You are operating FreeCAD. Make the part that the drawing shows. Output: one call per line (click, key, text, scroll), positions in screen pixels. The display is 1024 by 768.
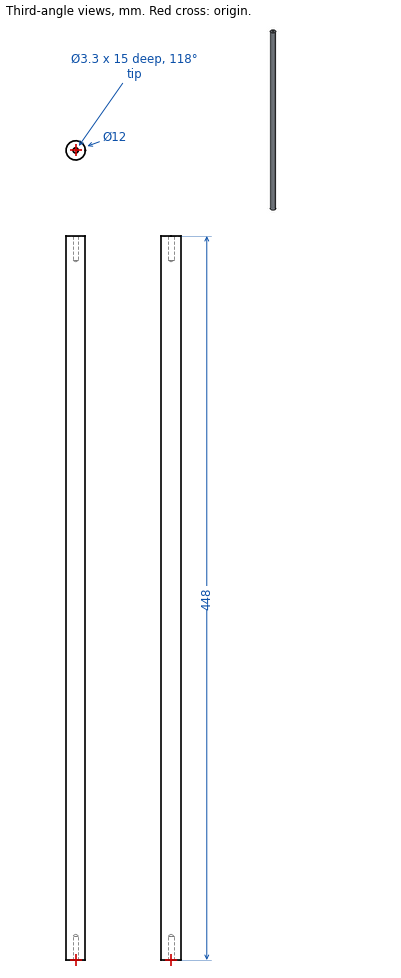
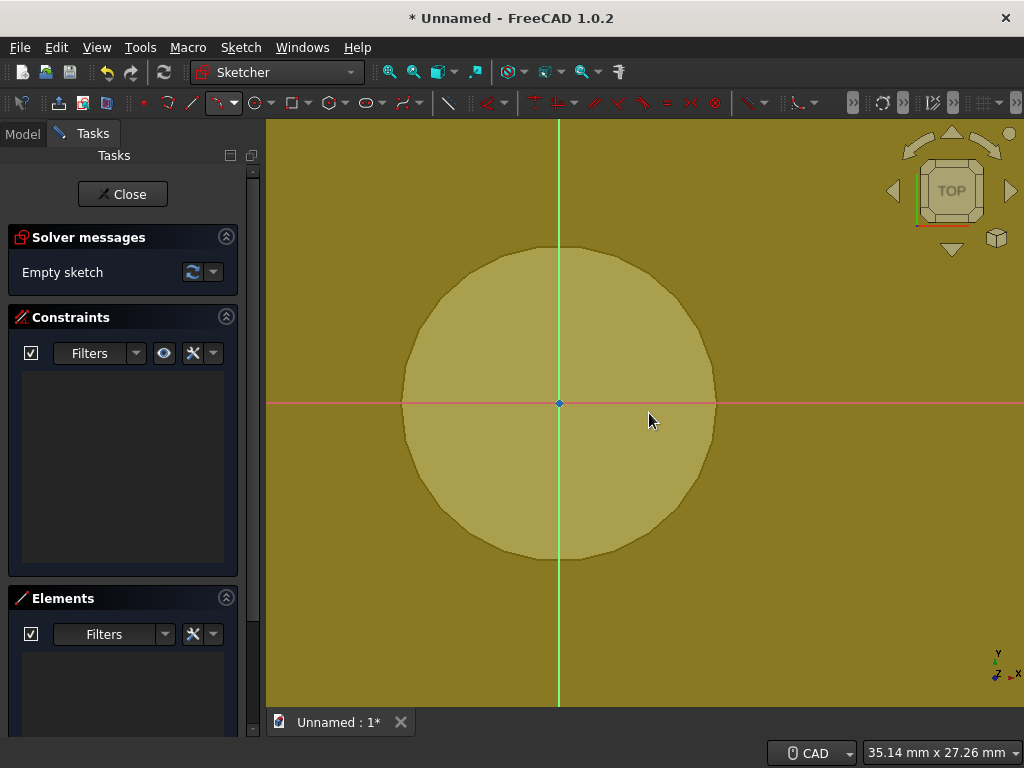
scroll(553, 400, up, 7)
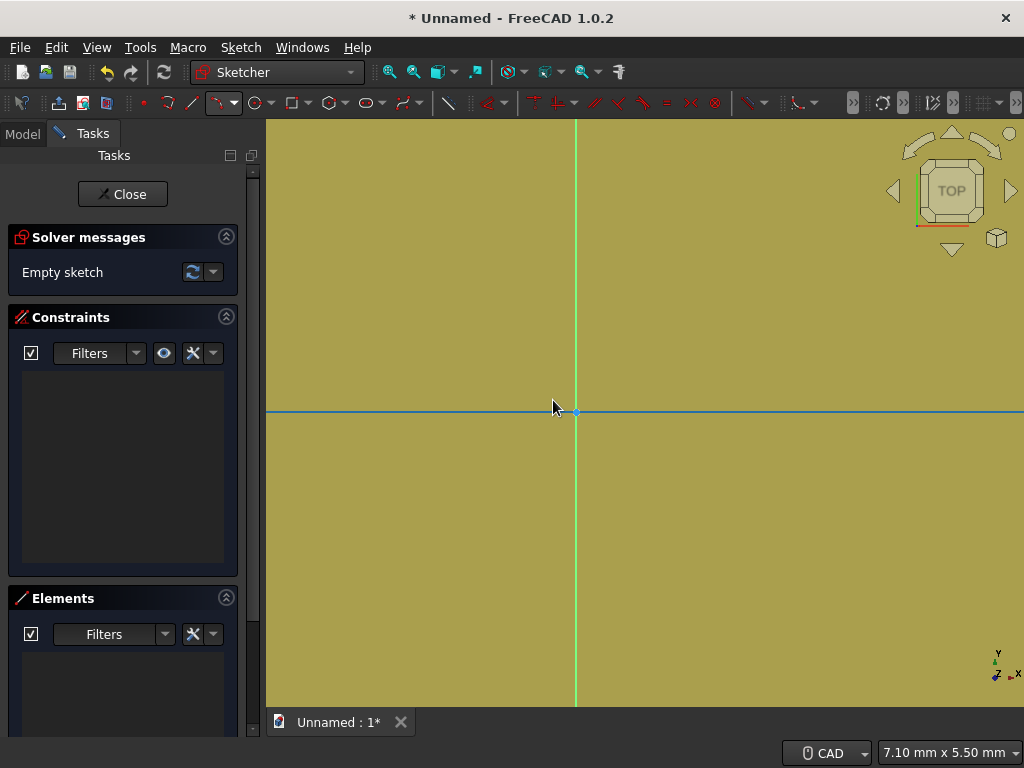
click(256, 104)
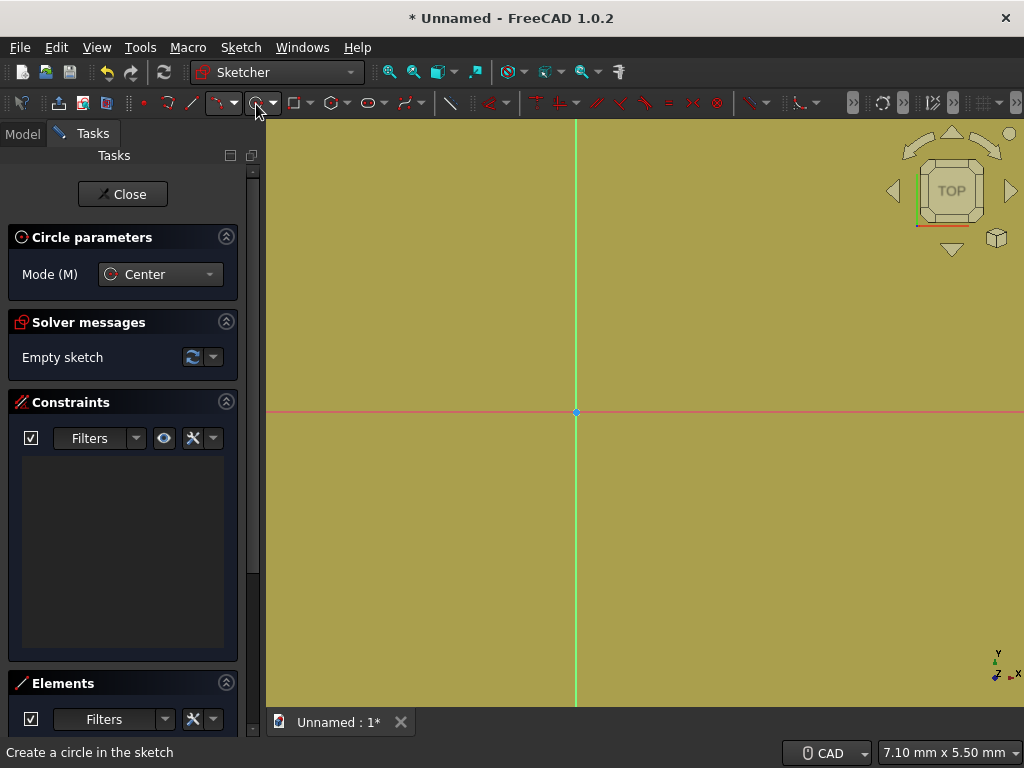
click(576, 412)
move(701, 288)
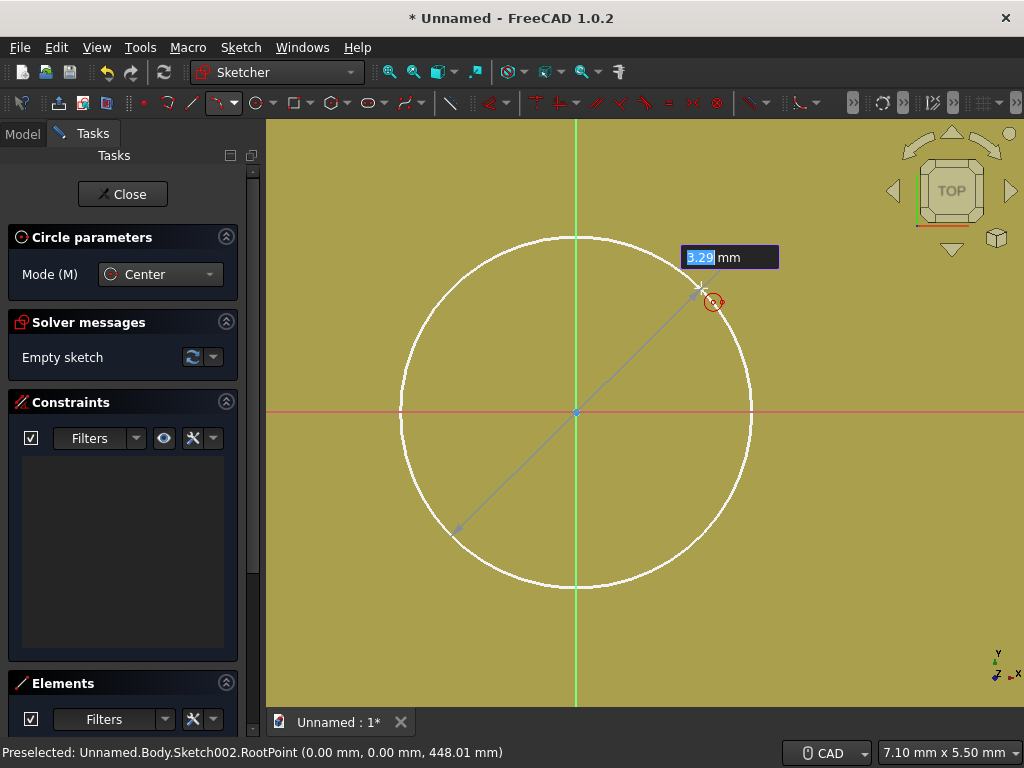
text(3.3)
key(Return)
key(Escape)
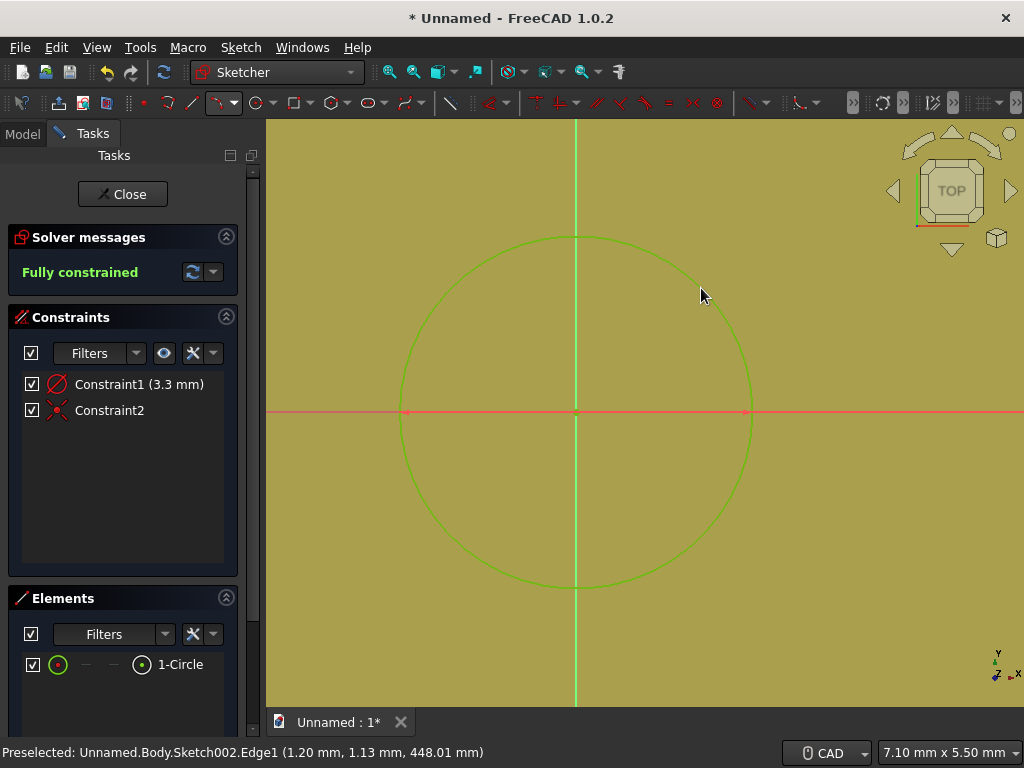
click(123, 194)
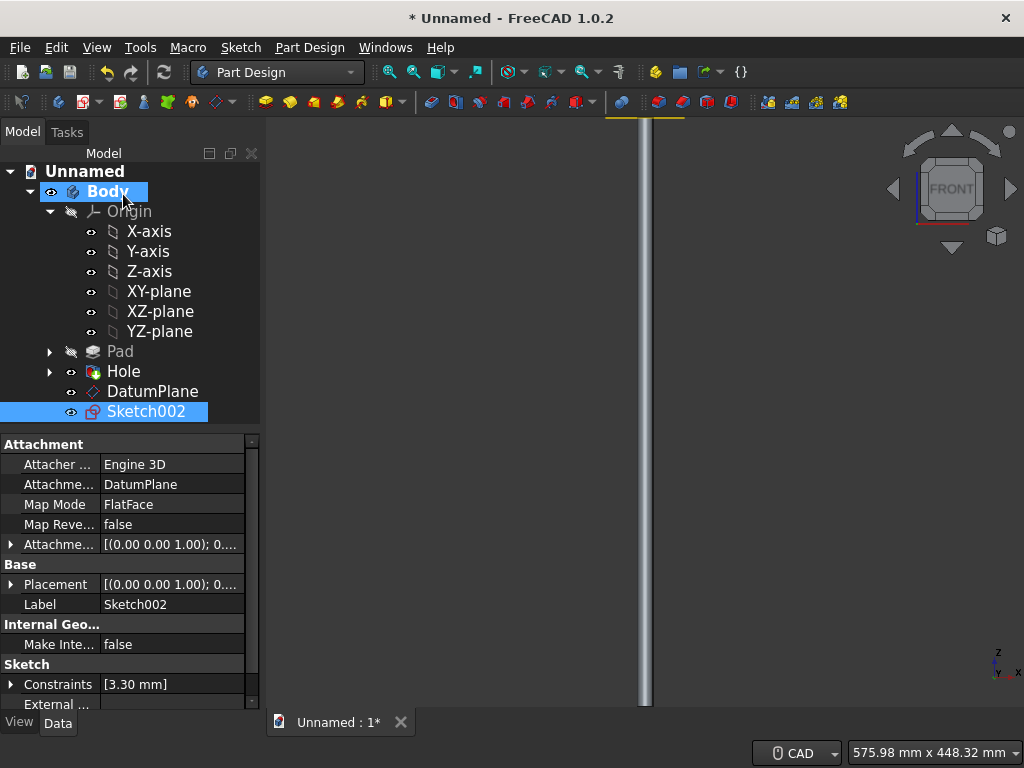
click(456, 102)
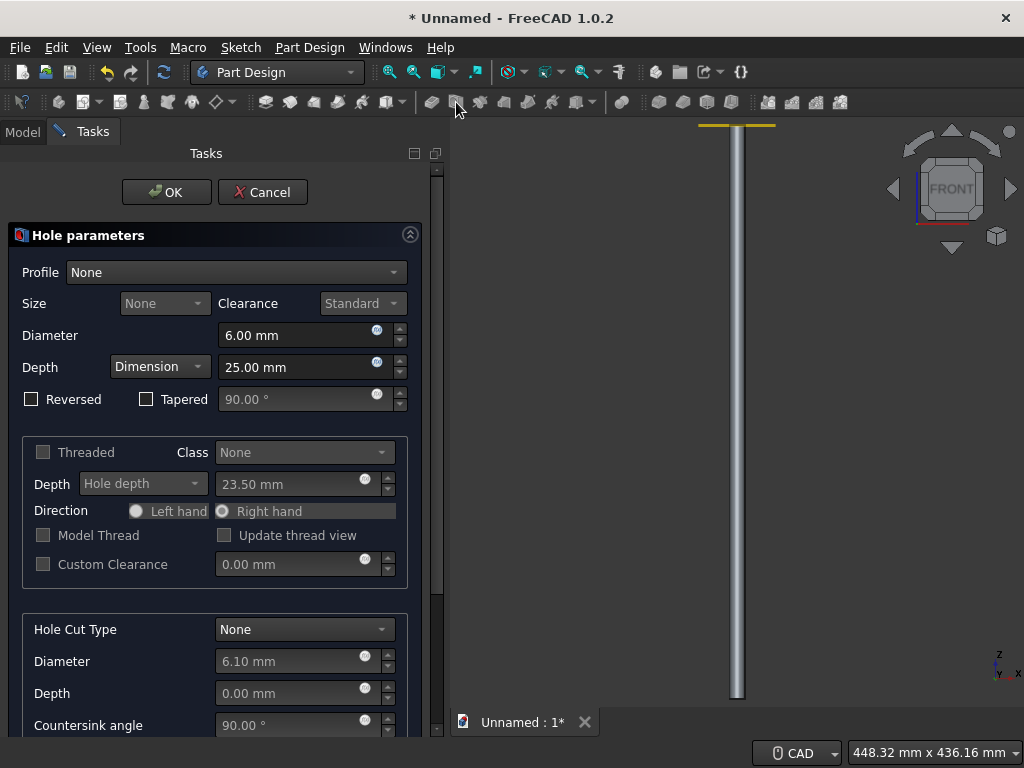
triple_click(305, 335)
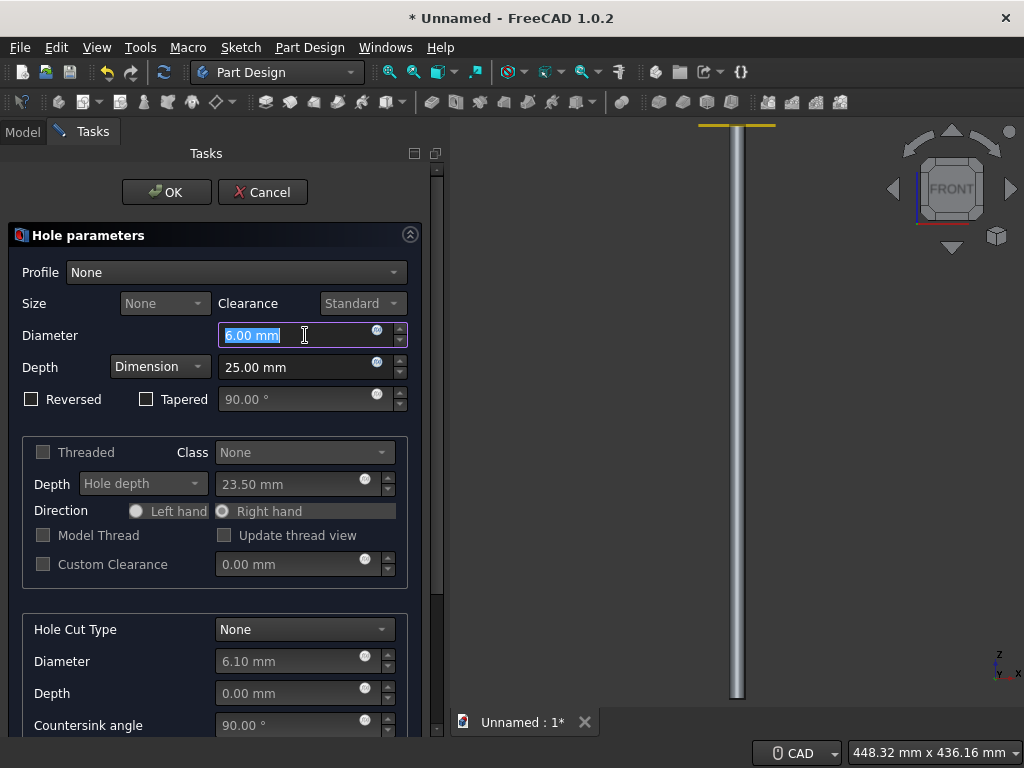
text(3.3)
key(Tab)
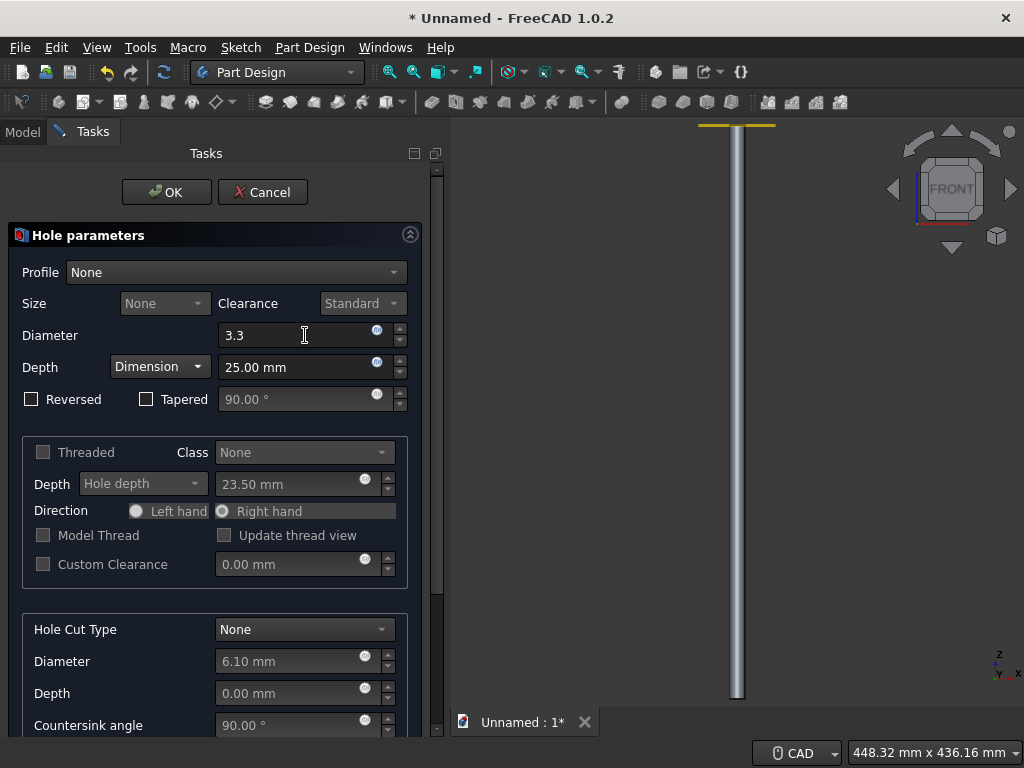
triple_click(305, 367)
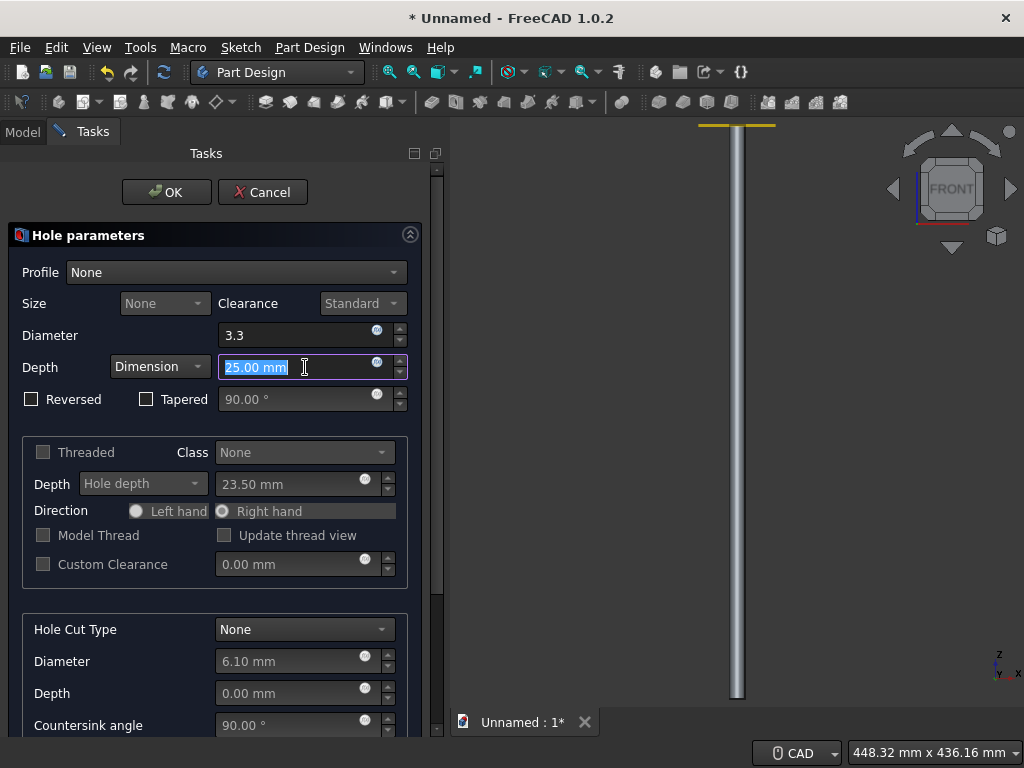
text(15)
key(Tab)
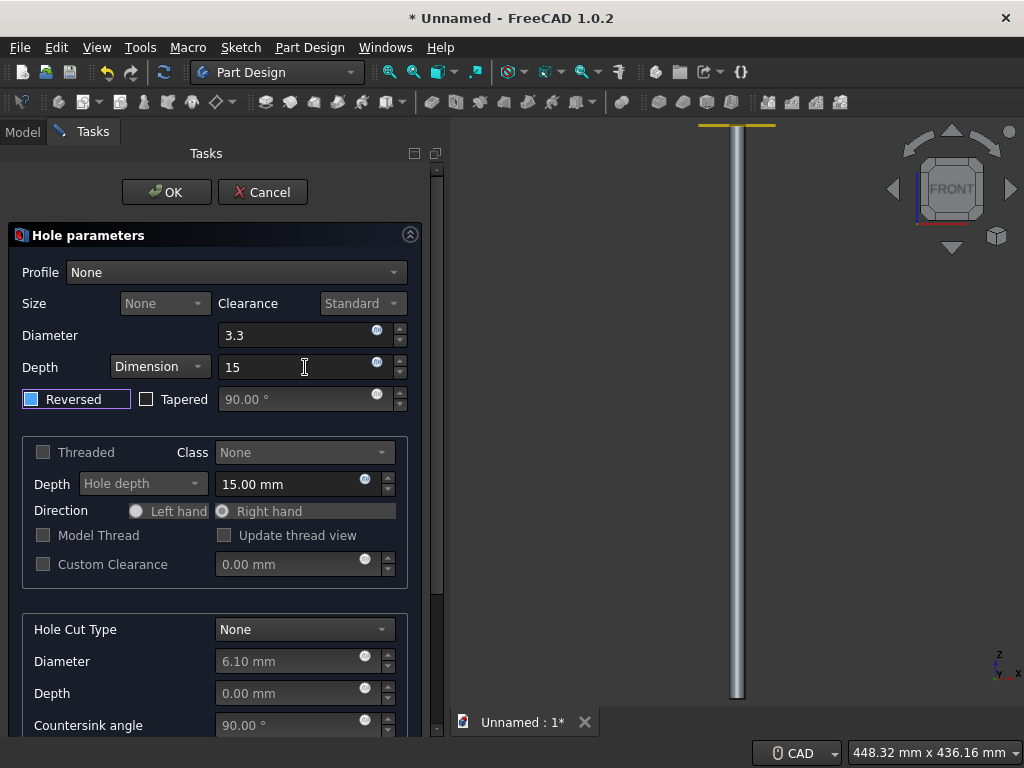
click(167, 192)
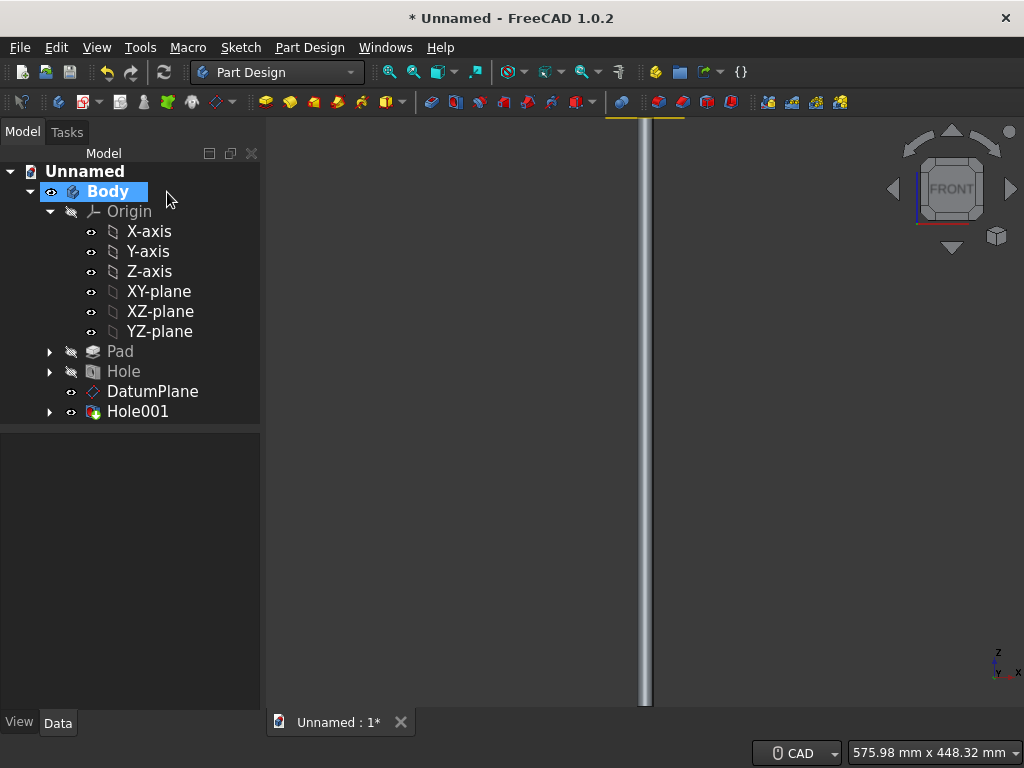
click(116, 392)
key(space)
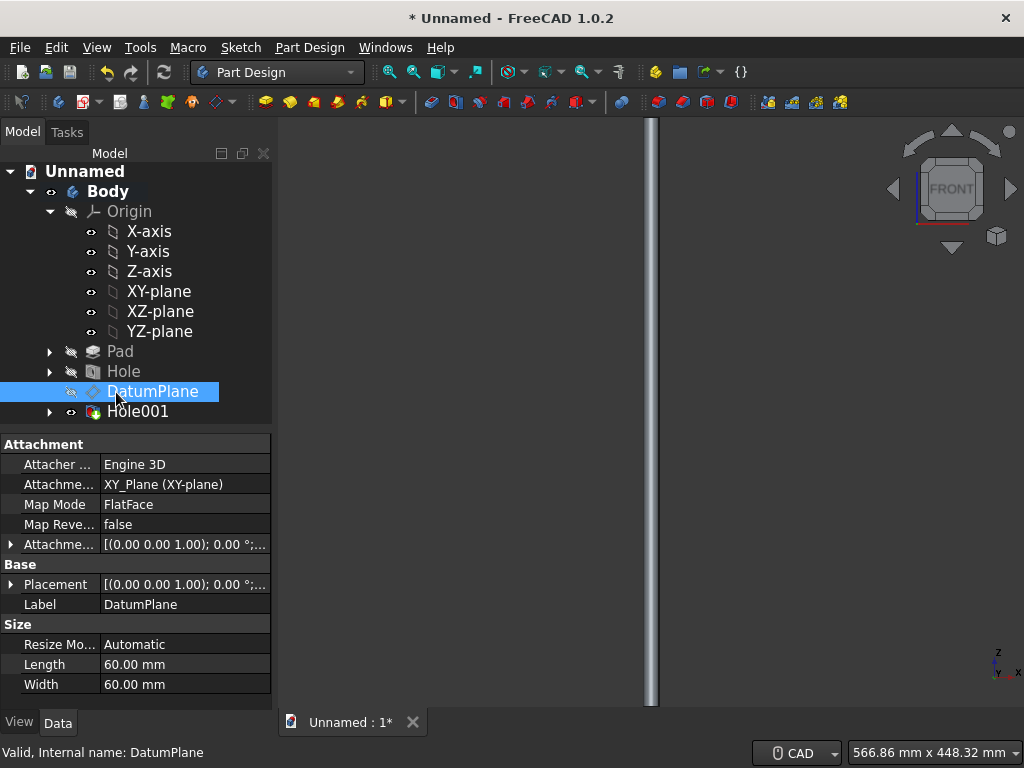
key(0)